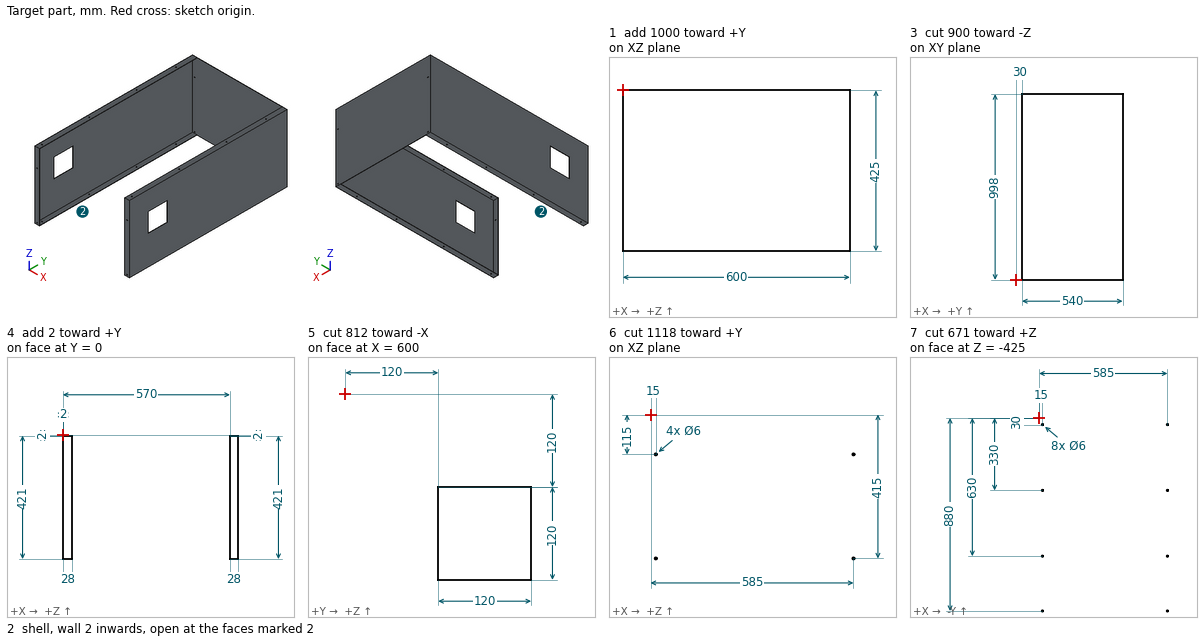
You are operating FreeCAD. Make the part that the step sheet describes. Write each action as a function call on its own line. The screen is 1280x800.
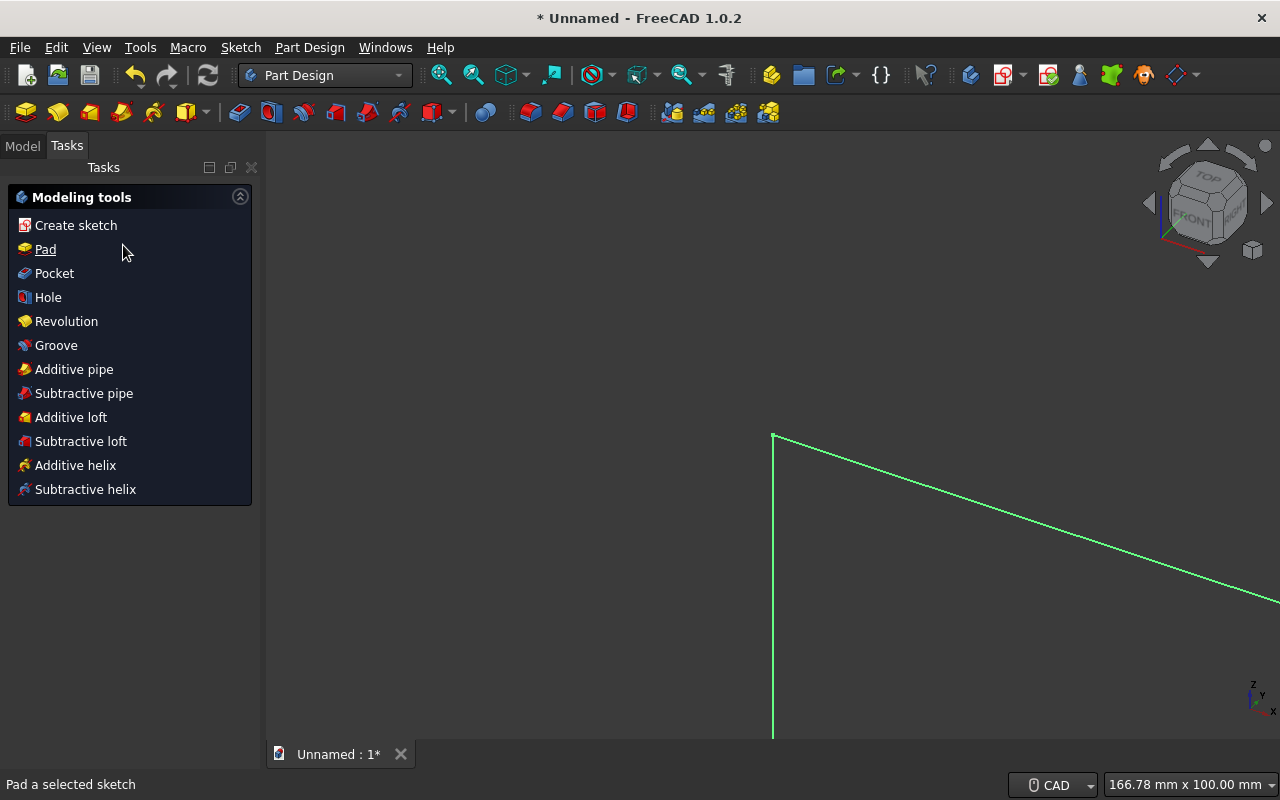
click(26, 112)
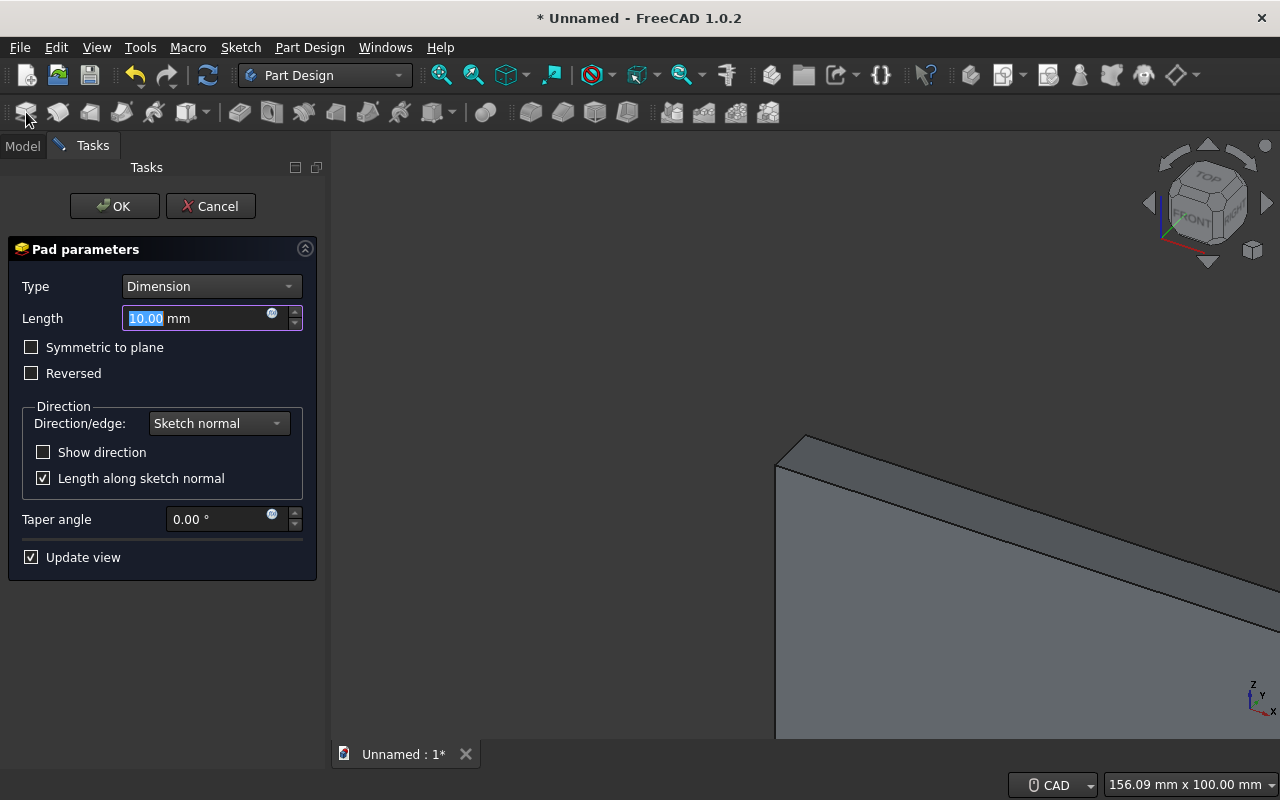
text(1000)
key(Tab)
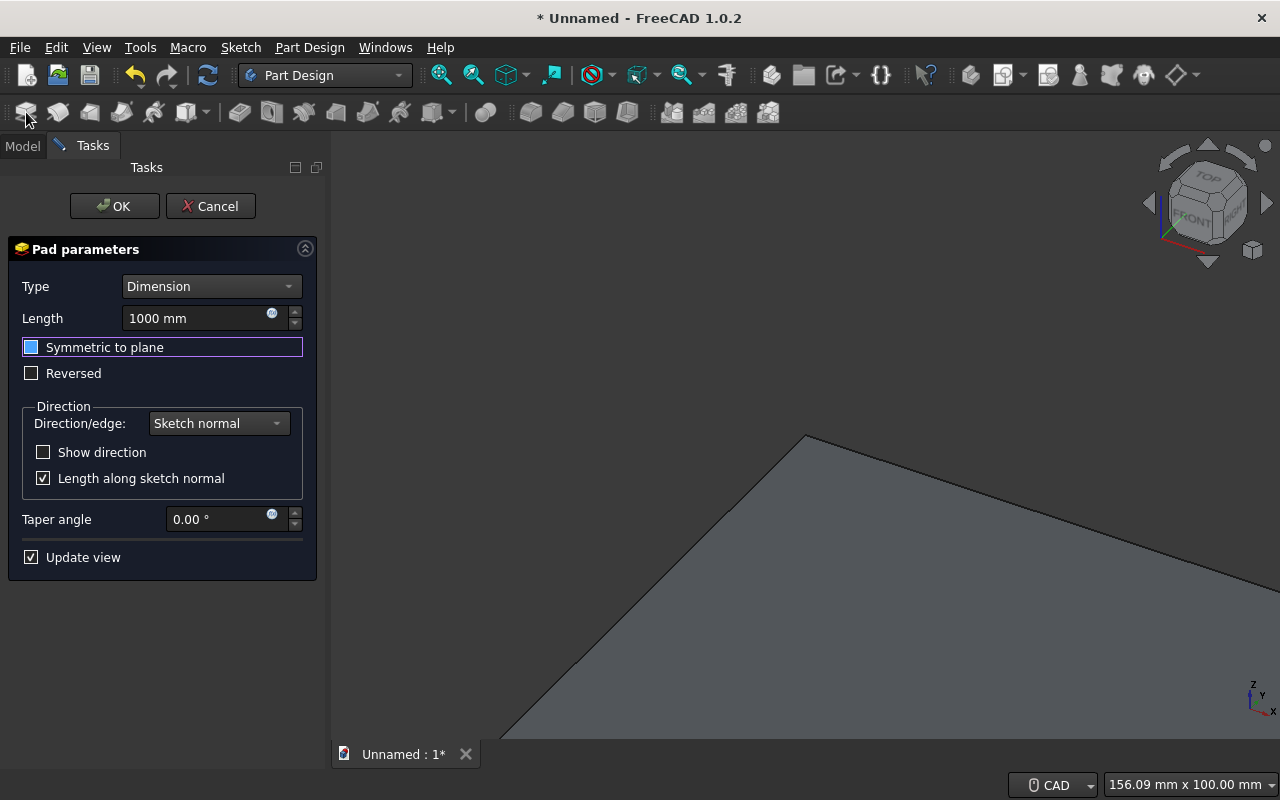
click(30, 373)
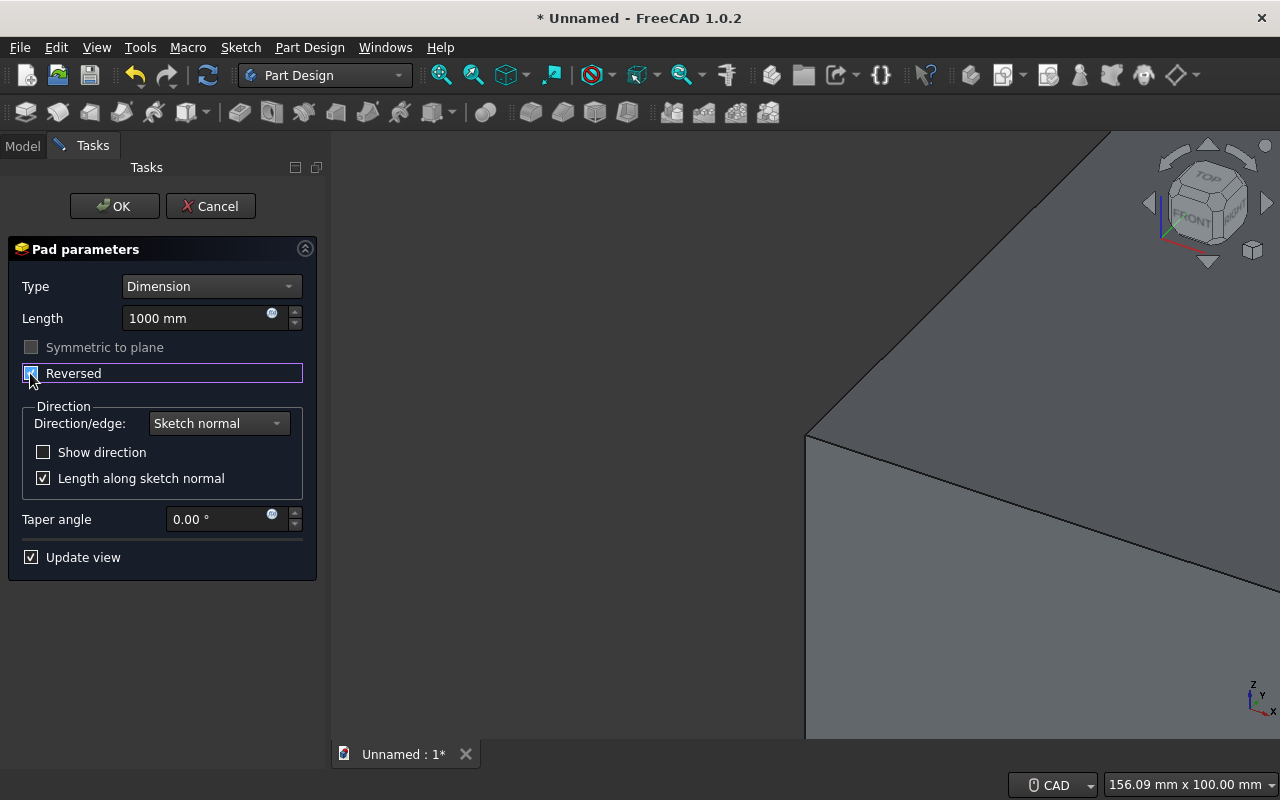
click(115, 206)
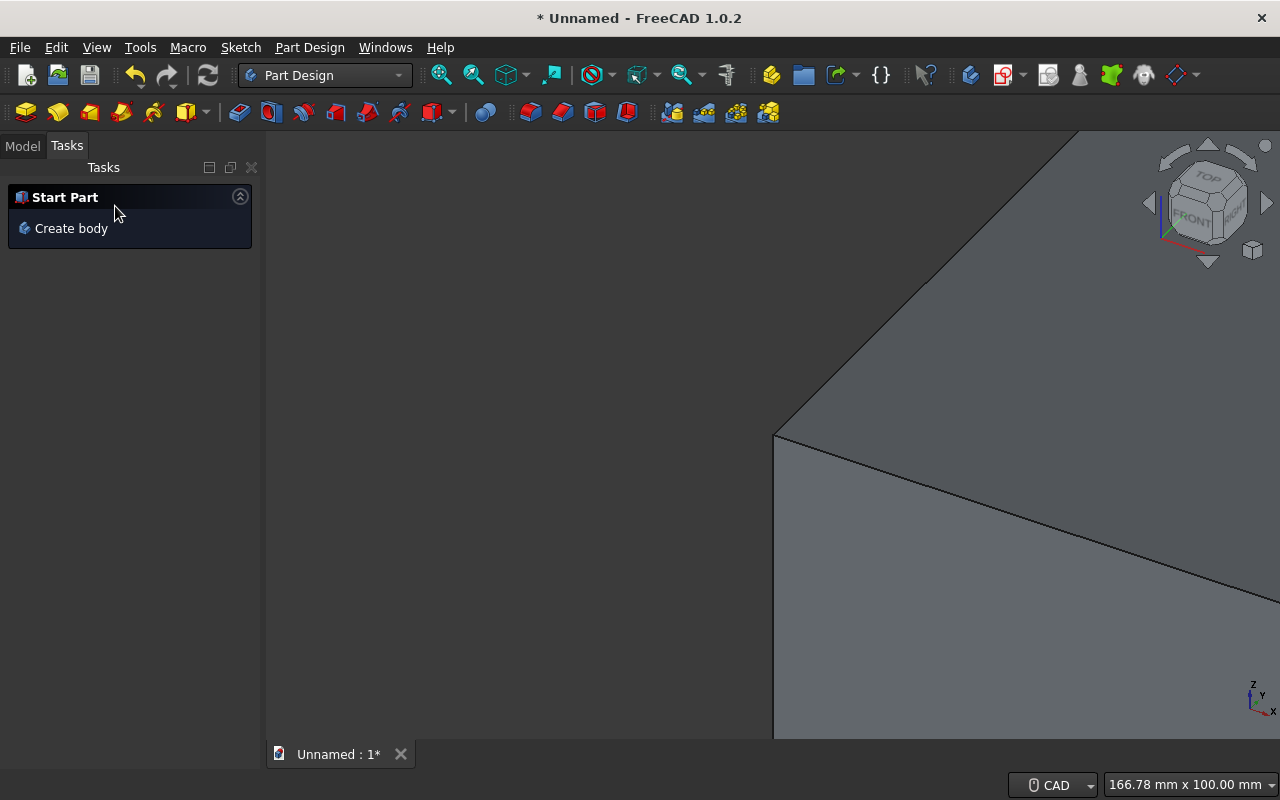
click(442, 76)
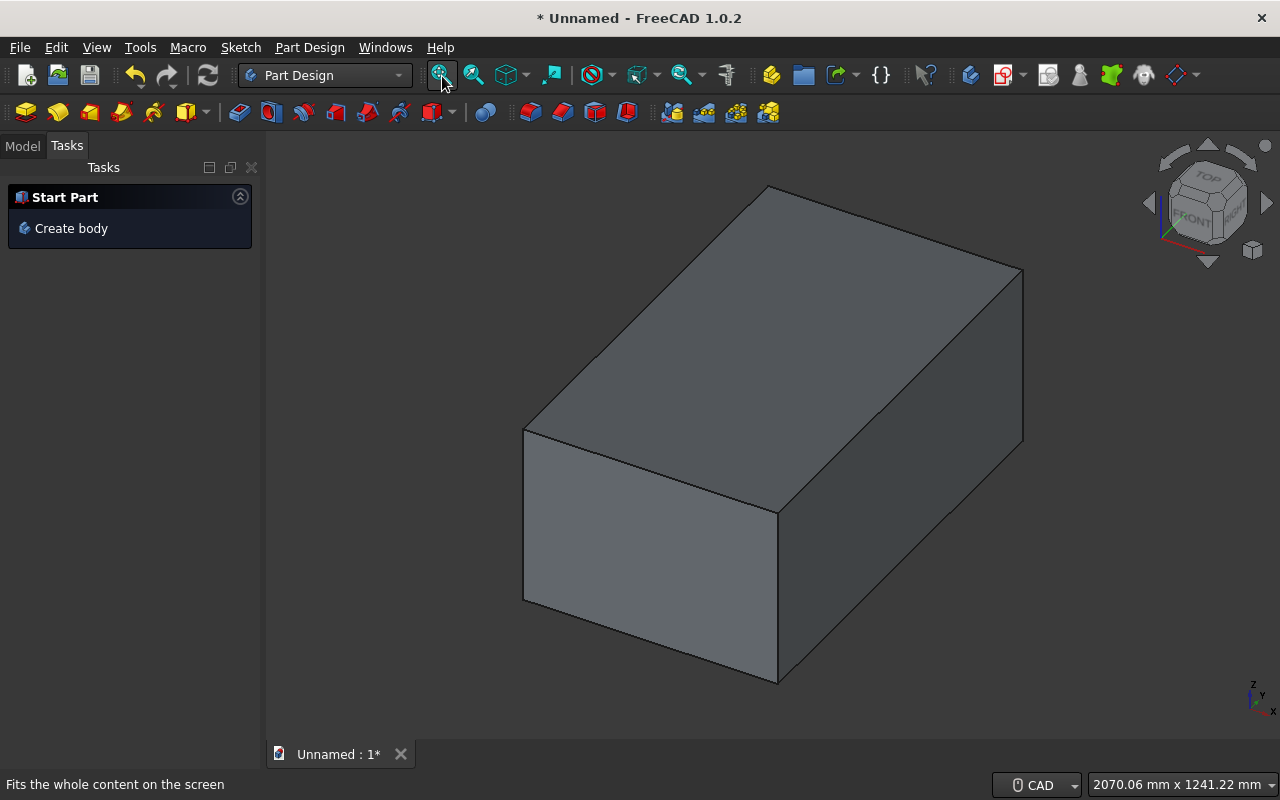
click(687, 568)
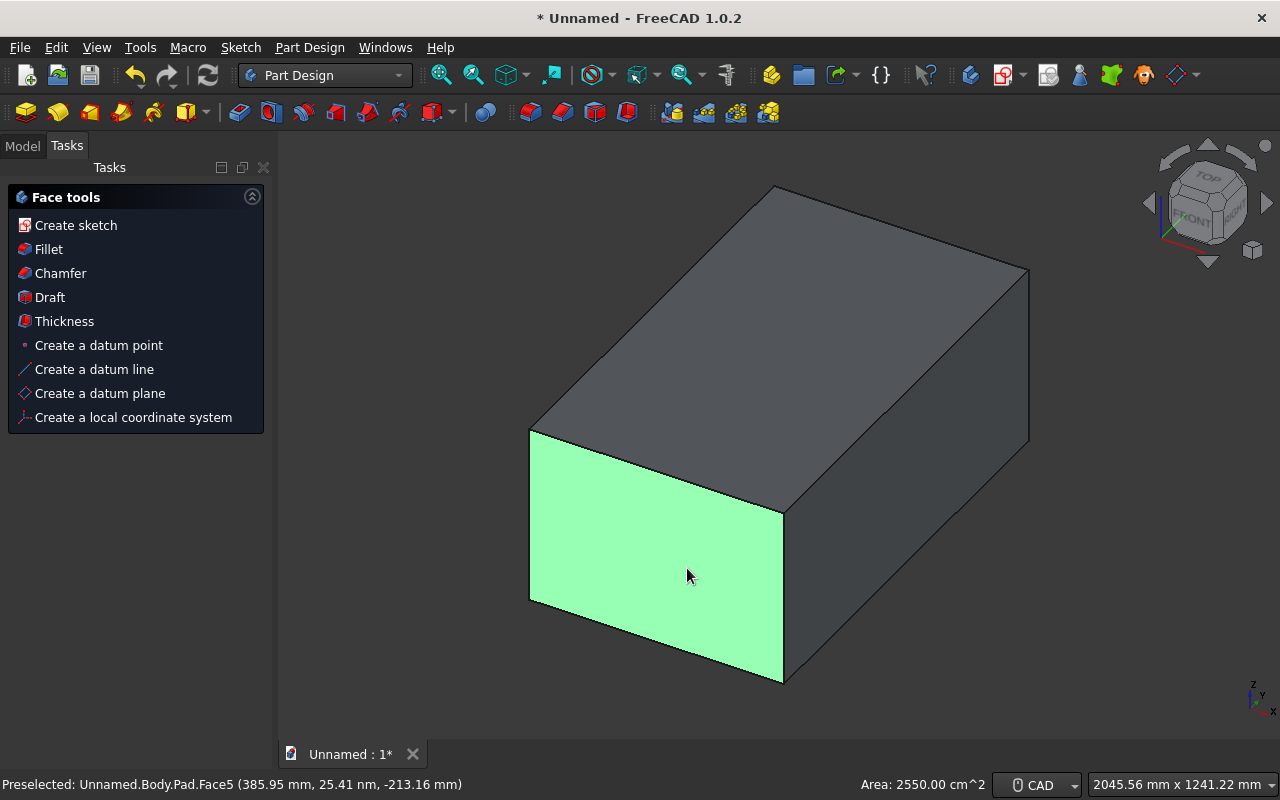
click(628, 112)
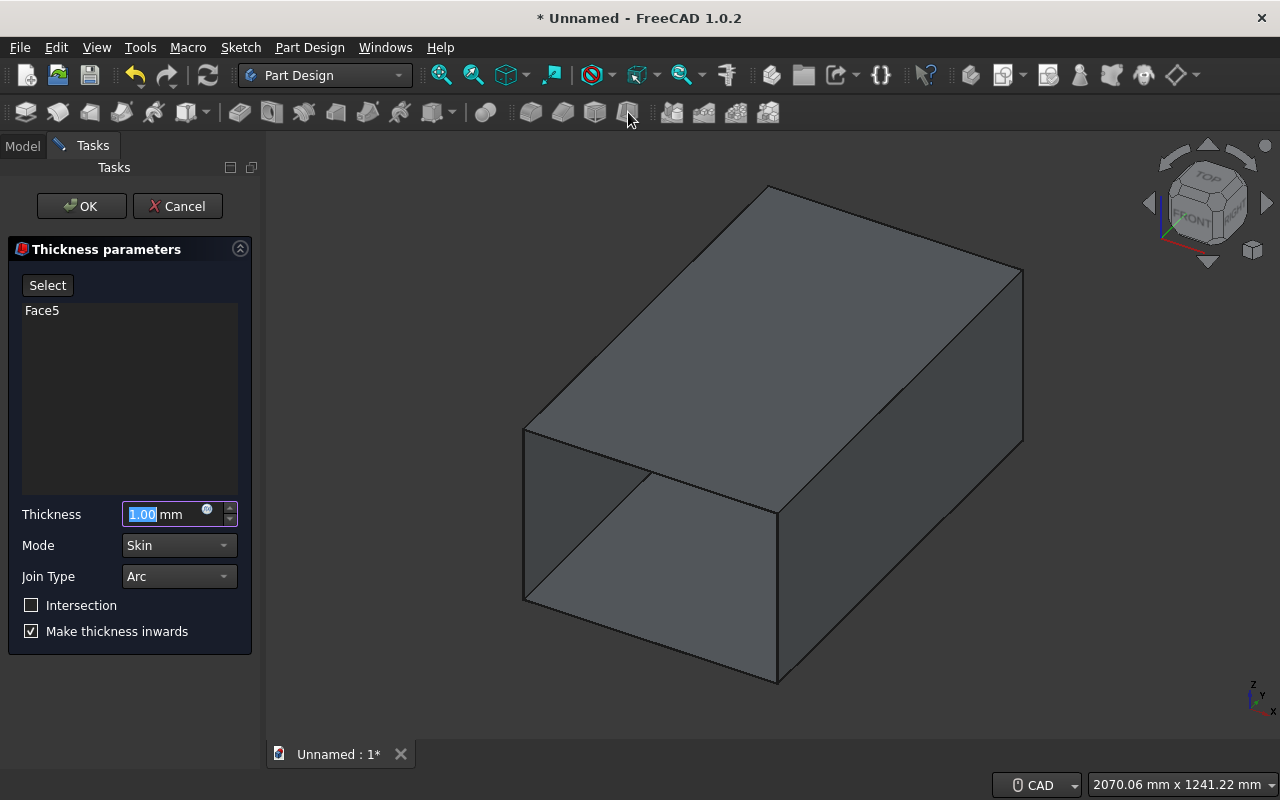
text(2)
key(Tab)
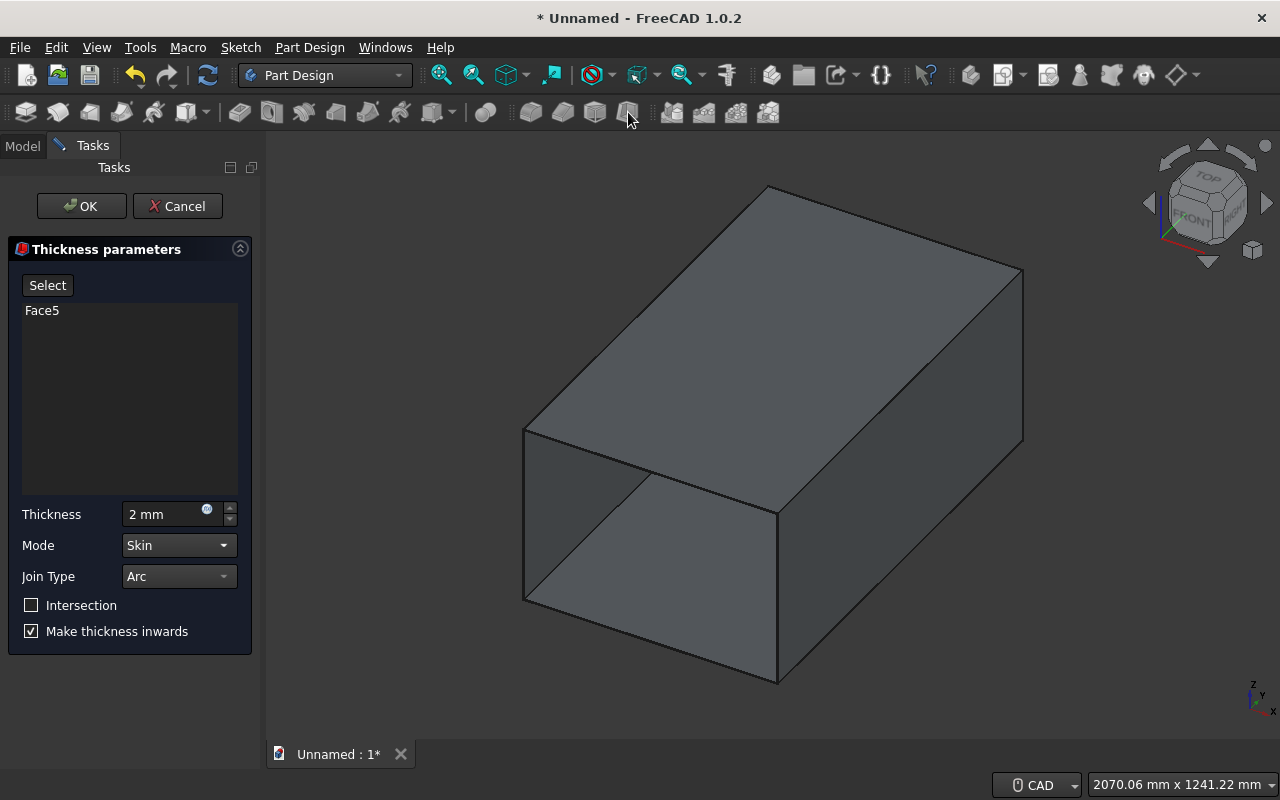
click(180, 576)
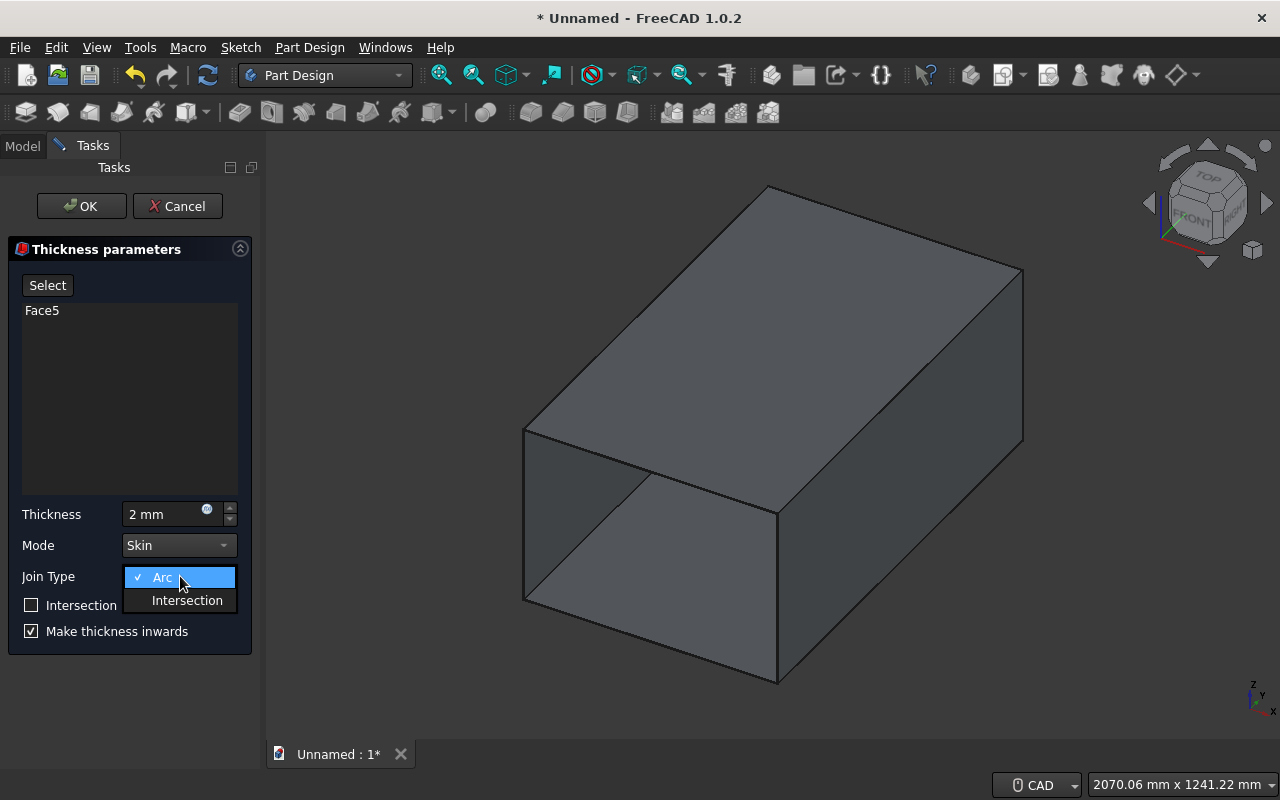
click(179, 600)